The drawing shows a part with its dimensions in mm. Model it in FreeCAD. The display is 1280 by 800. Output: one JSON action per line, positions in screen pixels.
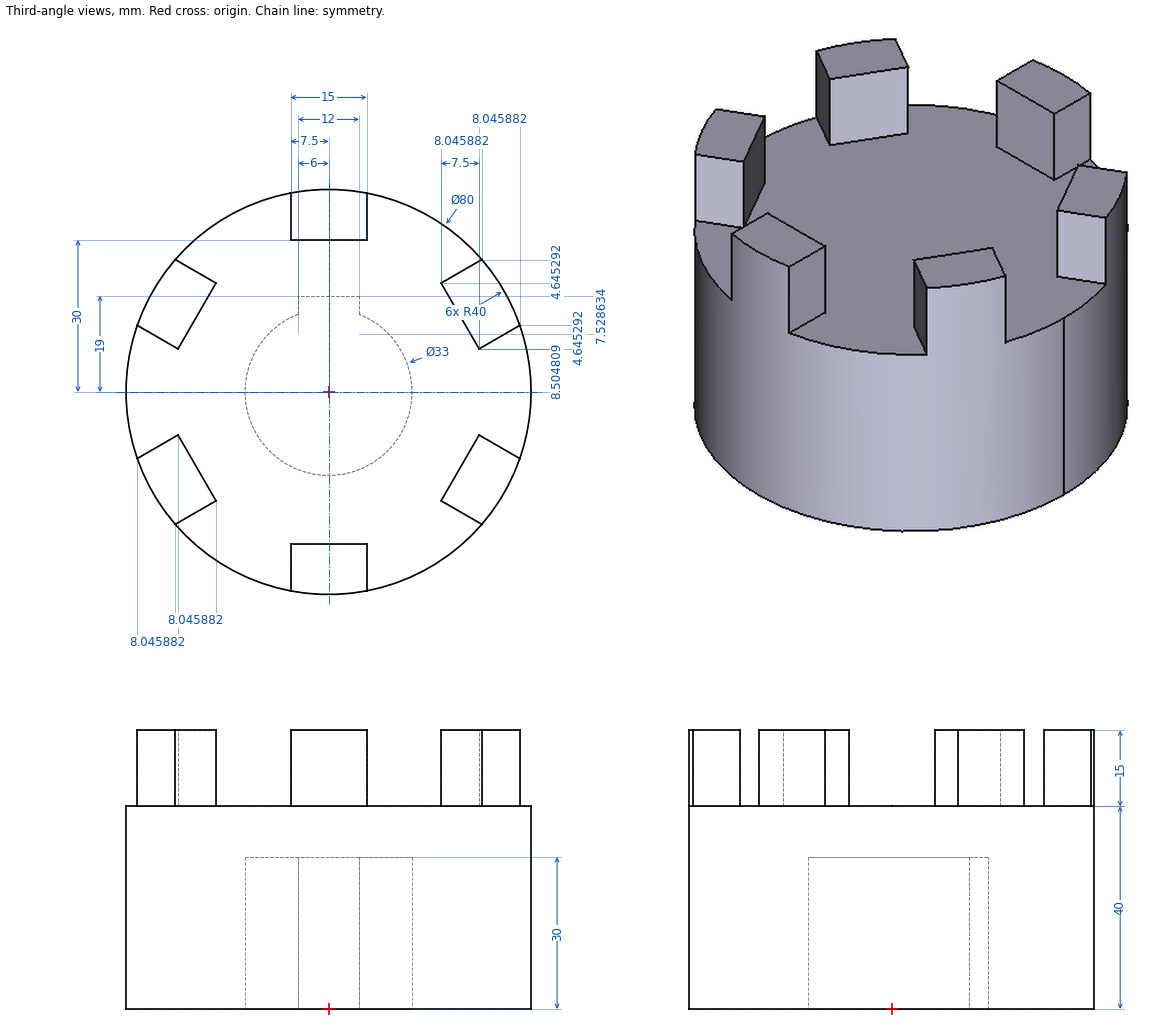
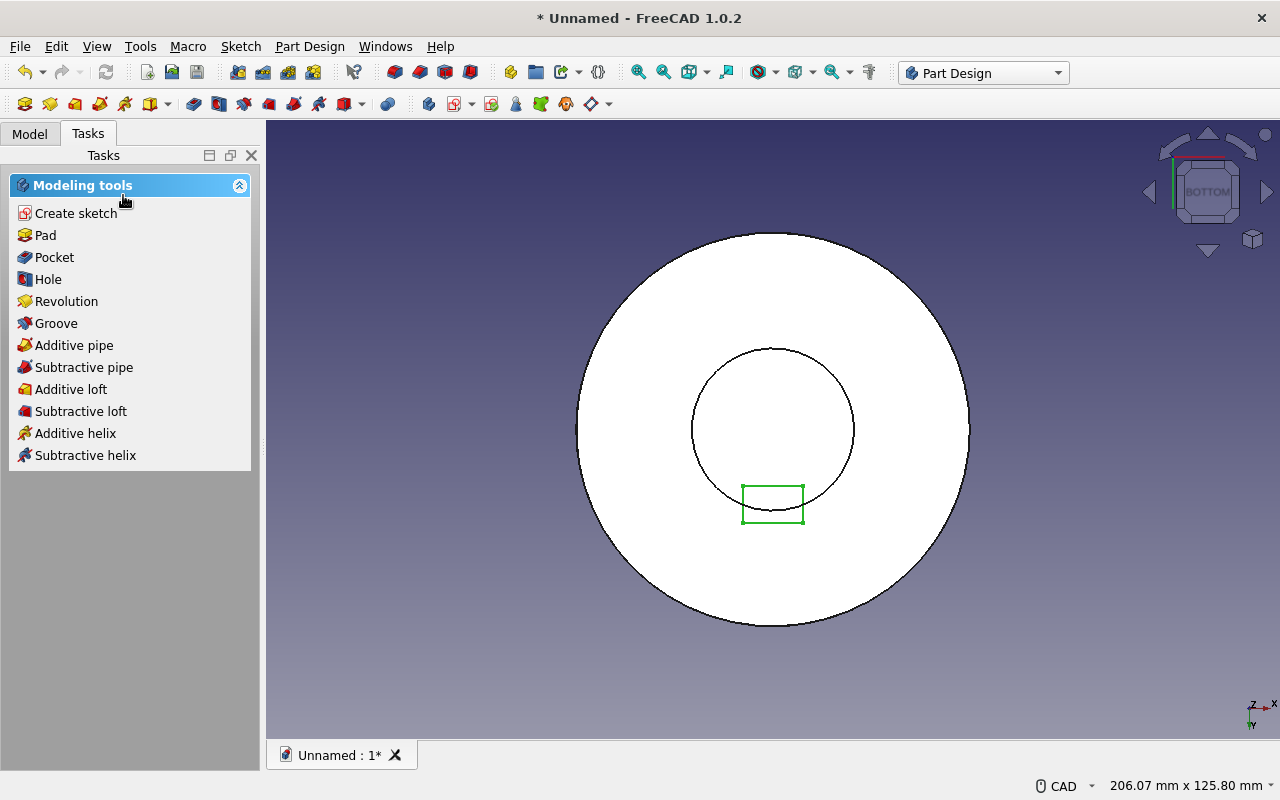
{"action": "left_click", "coordinate": [194, 104]}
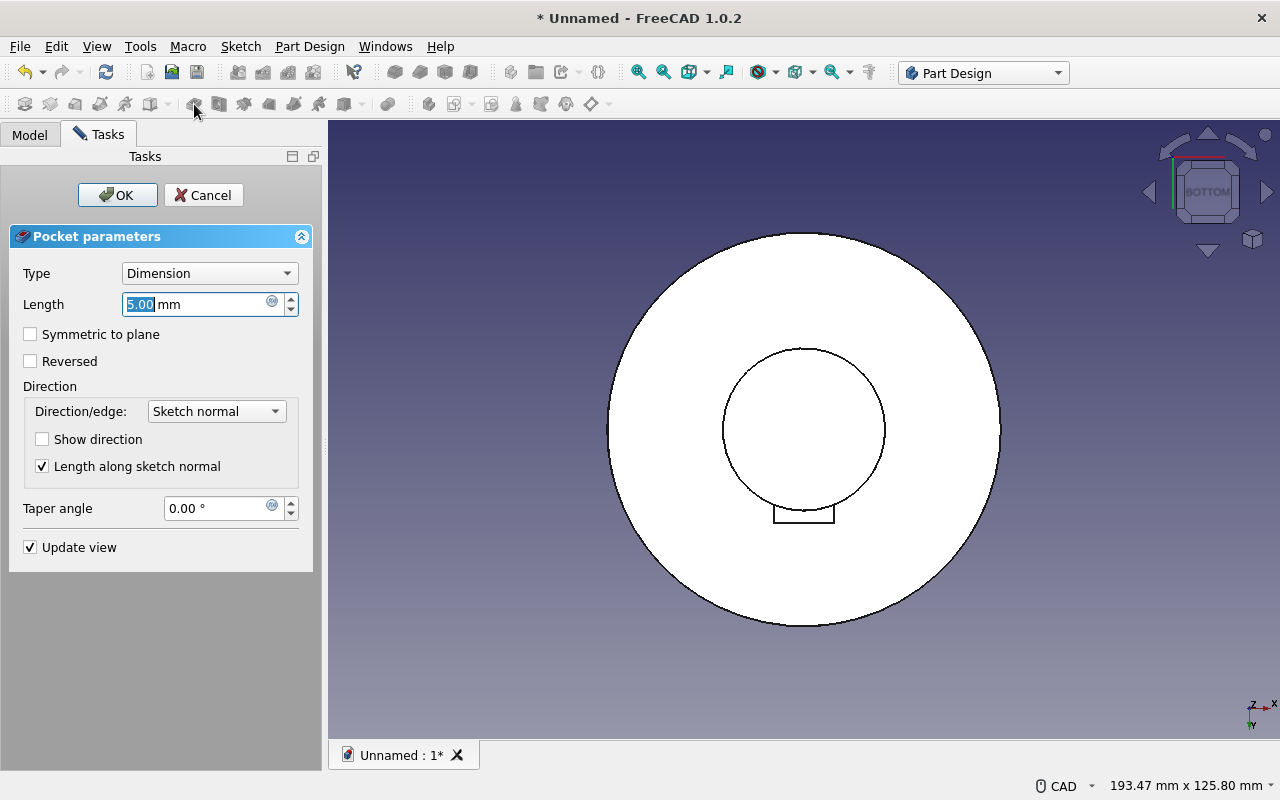
{"action": "type", "text": "30"}
{"action": "key", "text": "Tab"}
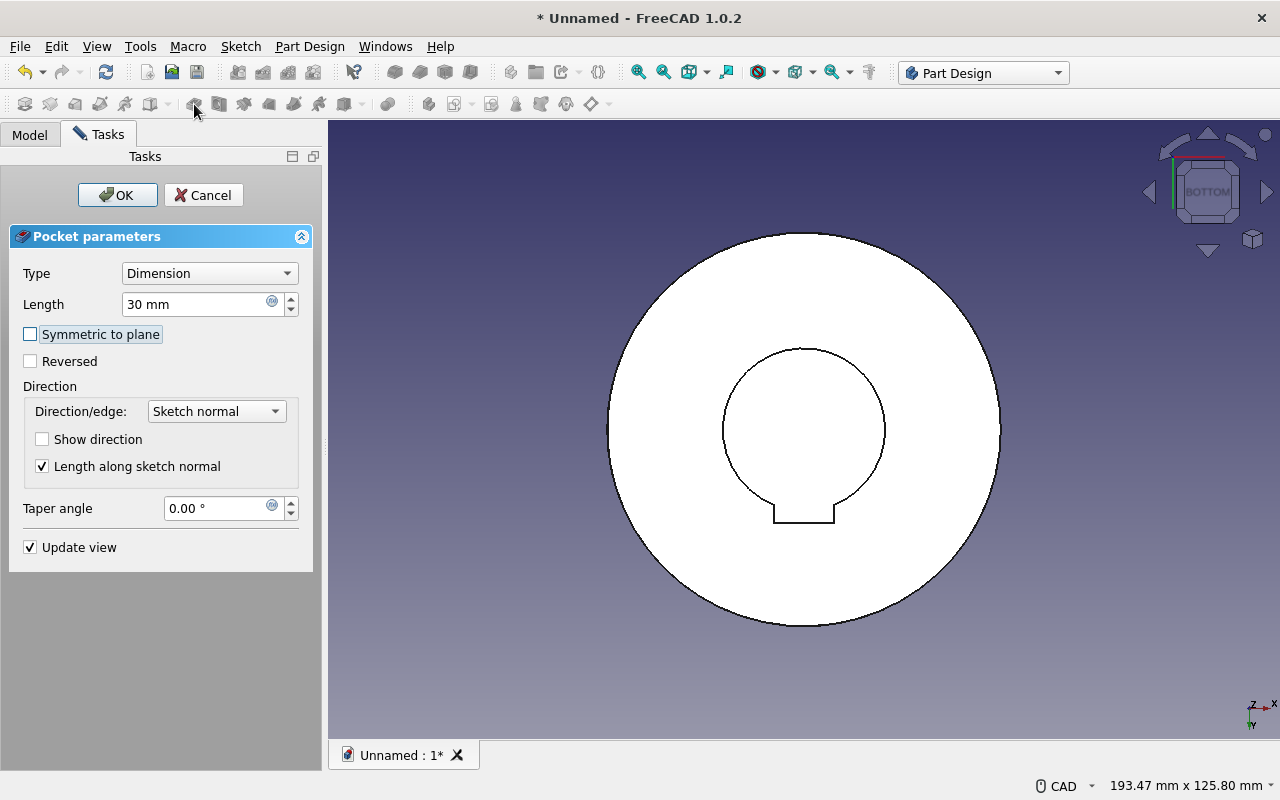
{"action": "left_click", "coordinate": [118, 195]}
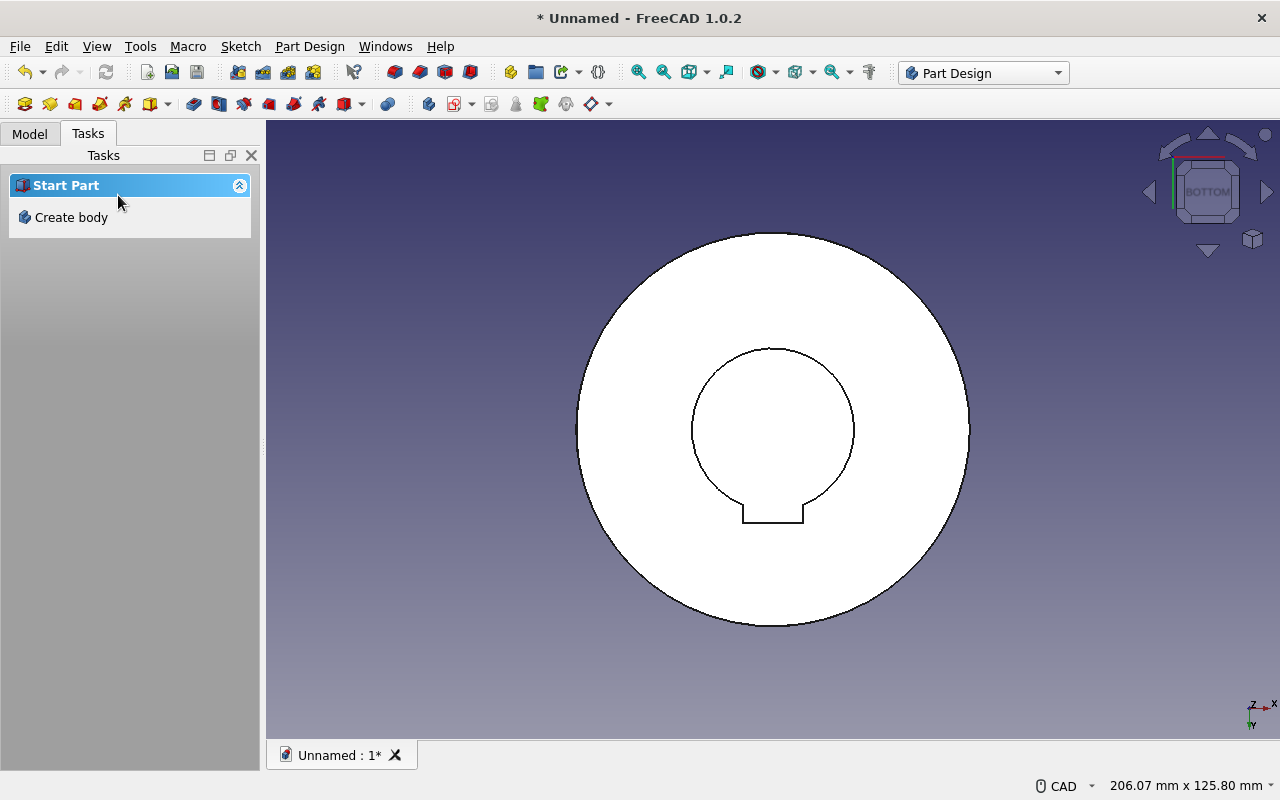
{"action": "key", "text": "0"}